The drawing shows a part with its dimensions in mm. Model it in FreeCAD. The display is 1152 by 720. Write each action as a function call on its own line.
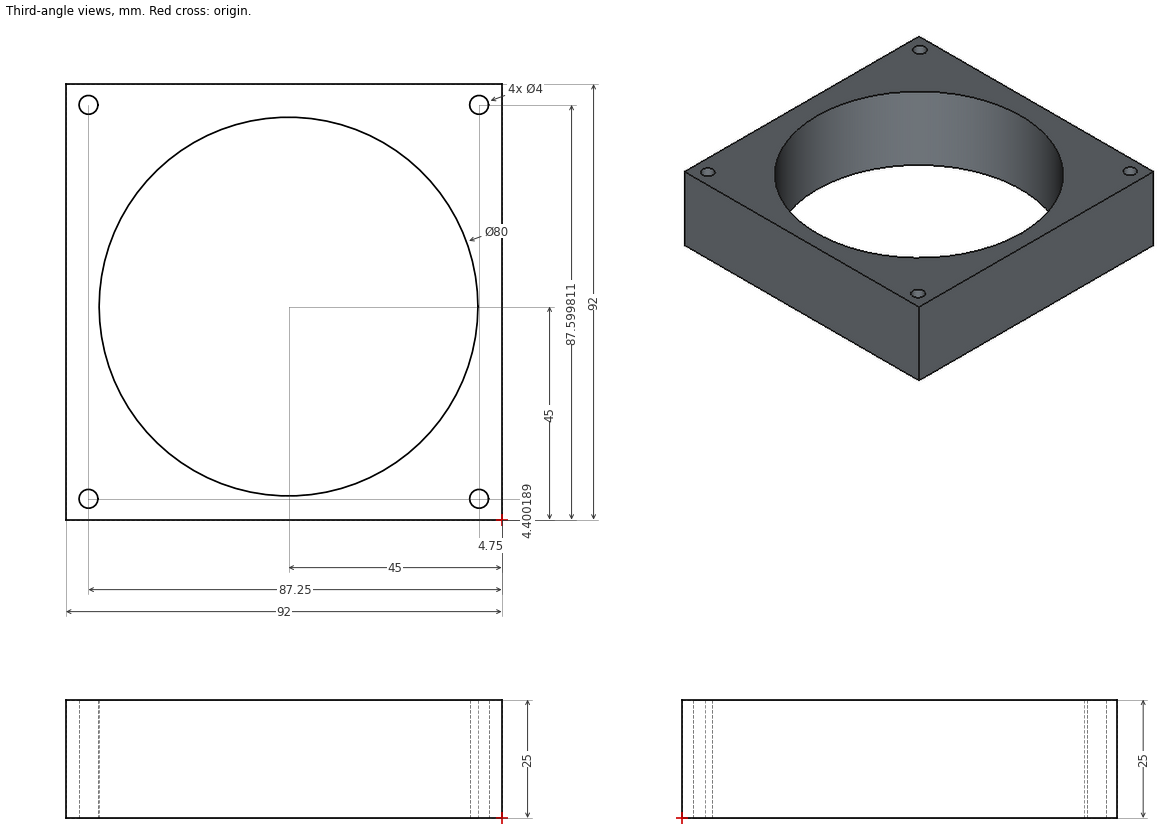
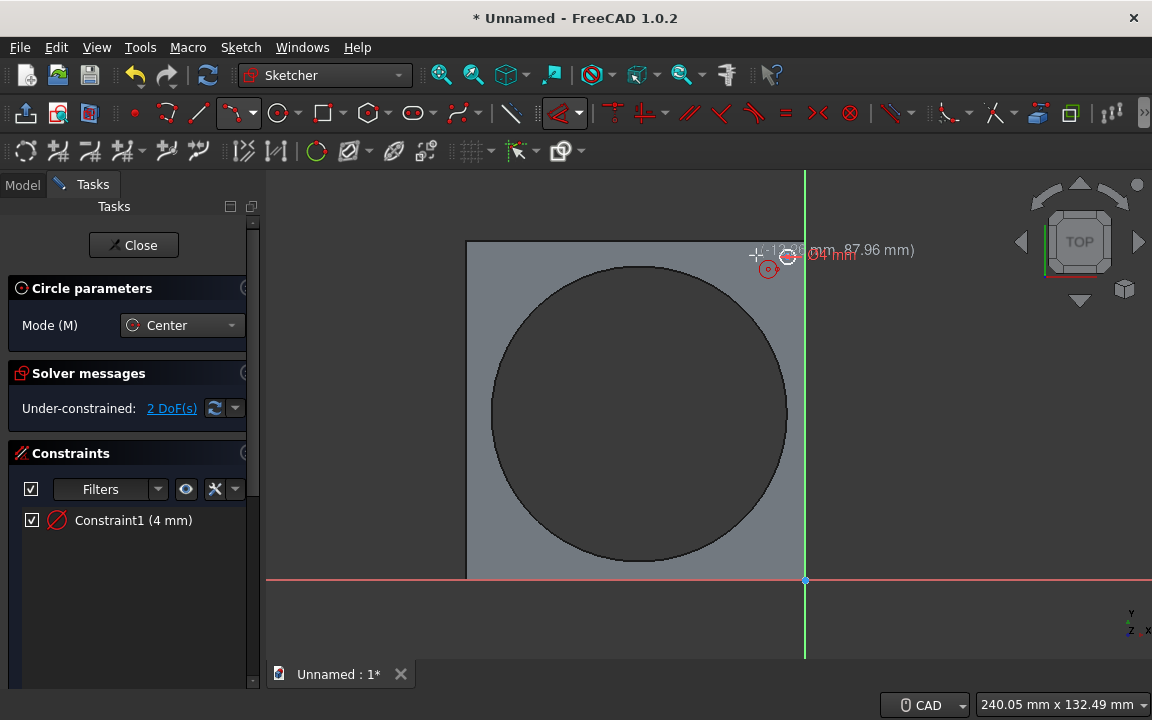
scroll(483, 257, up, 6)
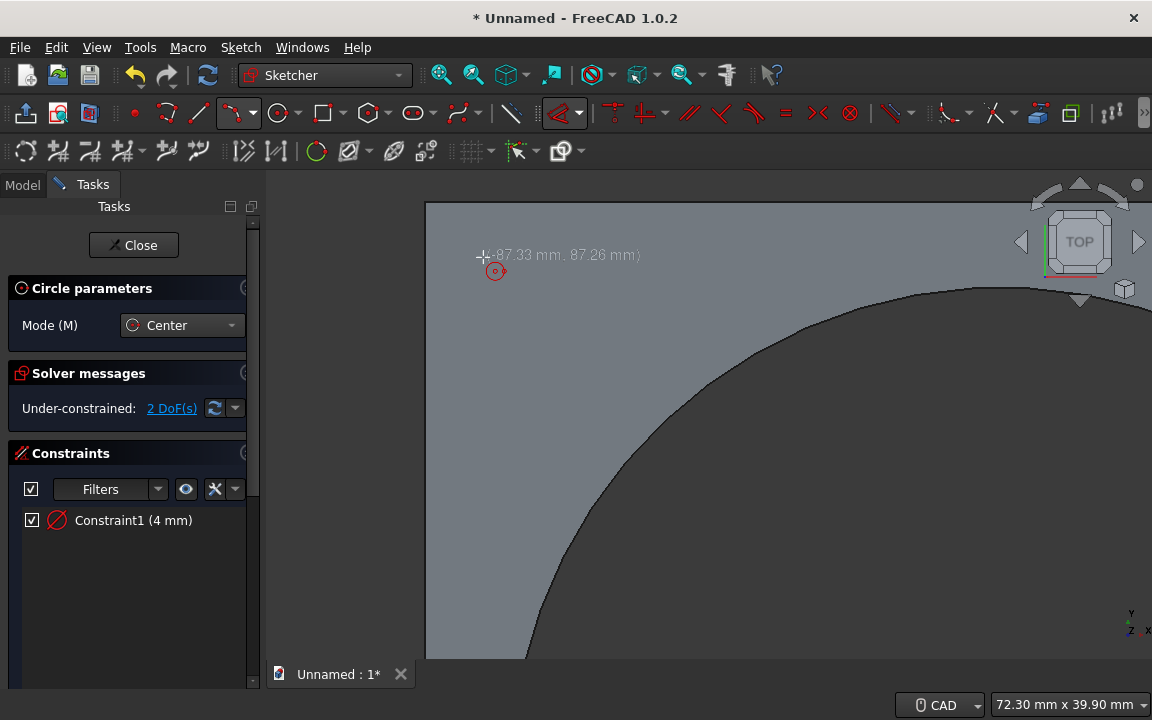
click(483, 256)
move(501, 238)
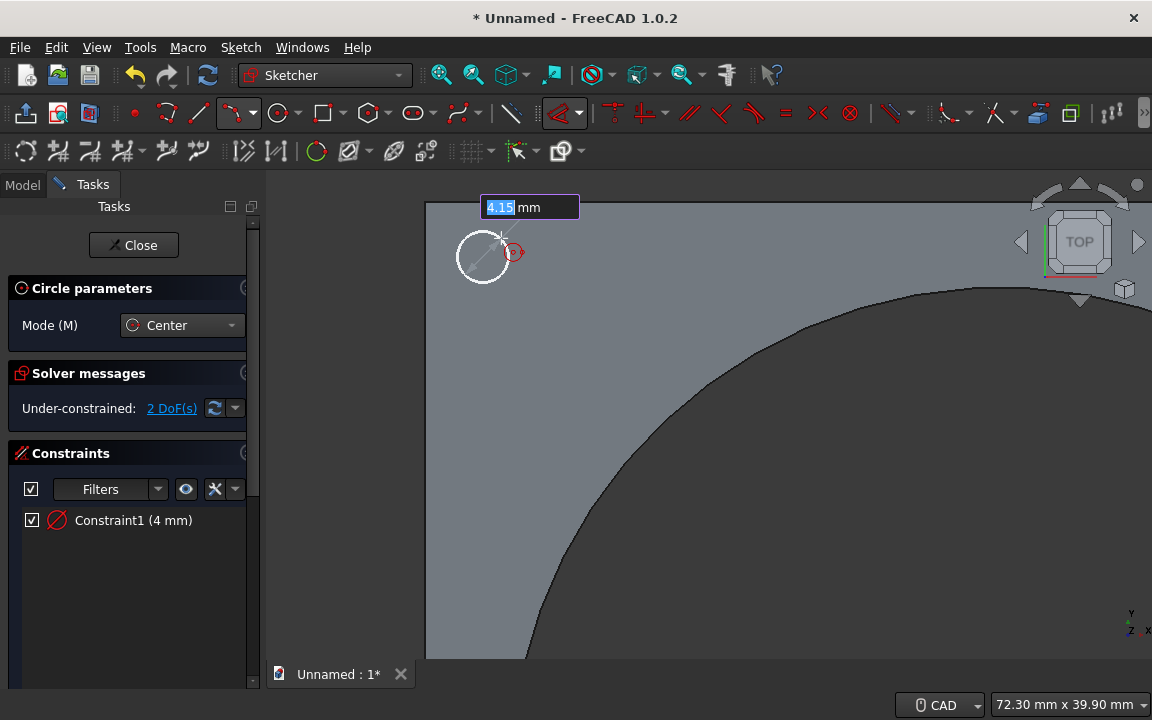
text(4)
key(Return)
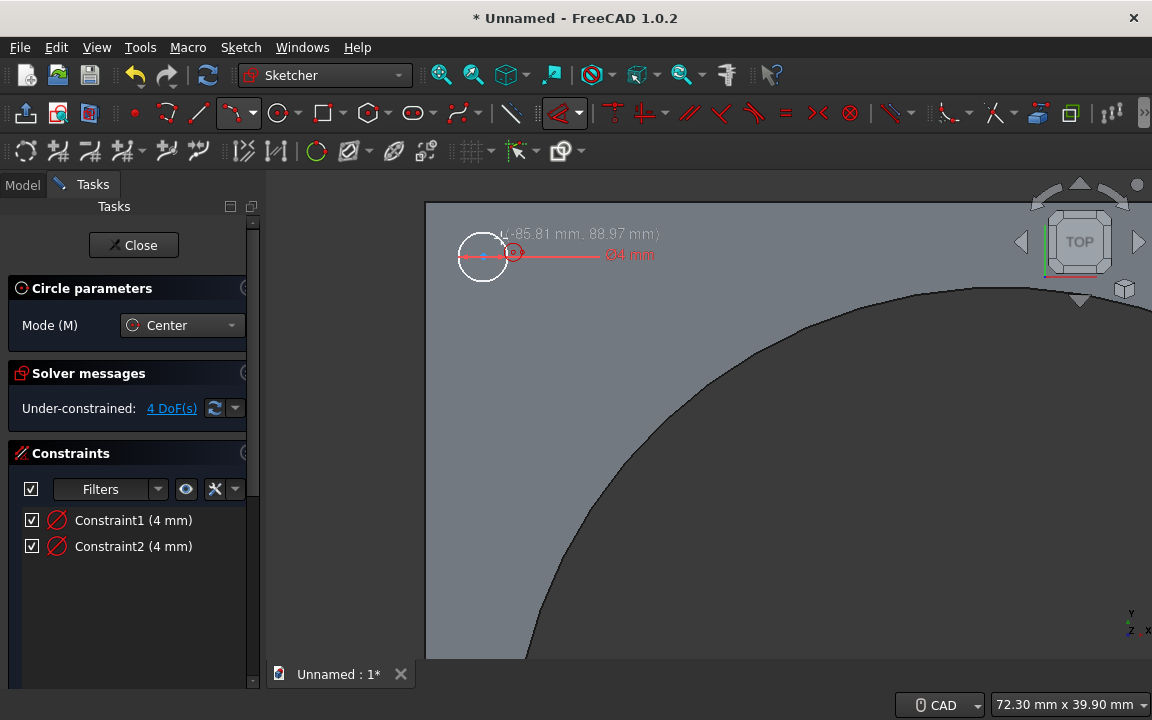
scroll(483, 257, down, 6)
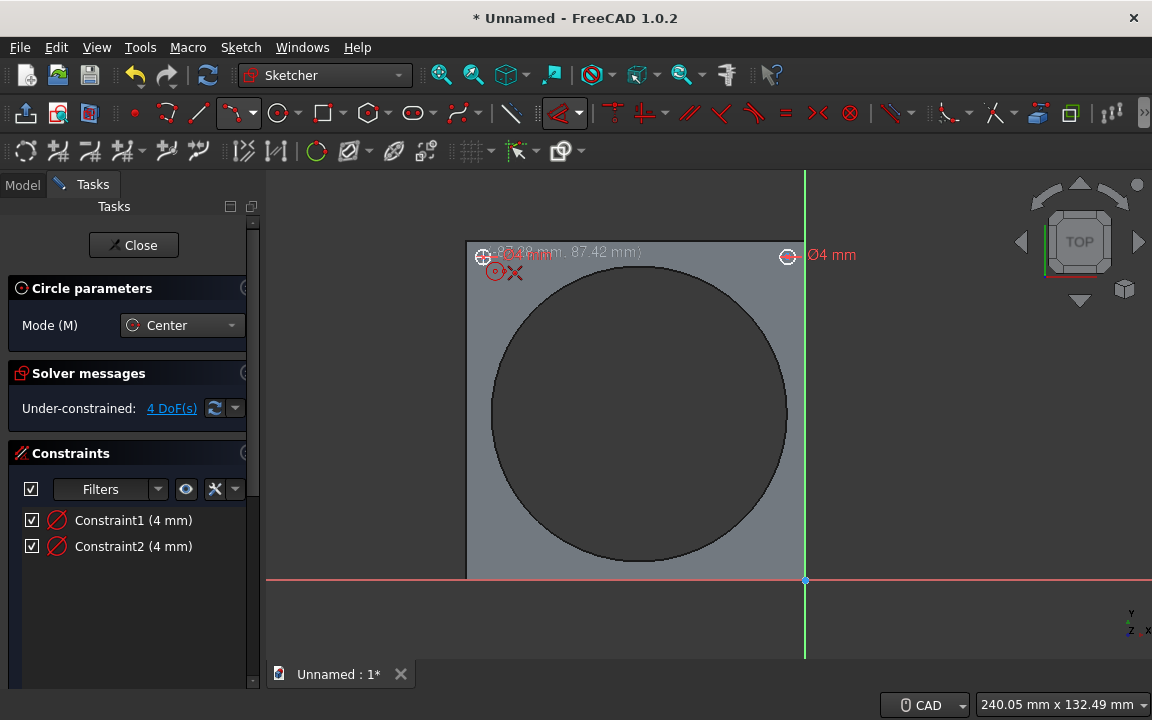
scroll(483, 564, up, 6)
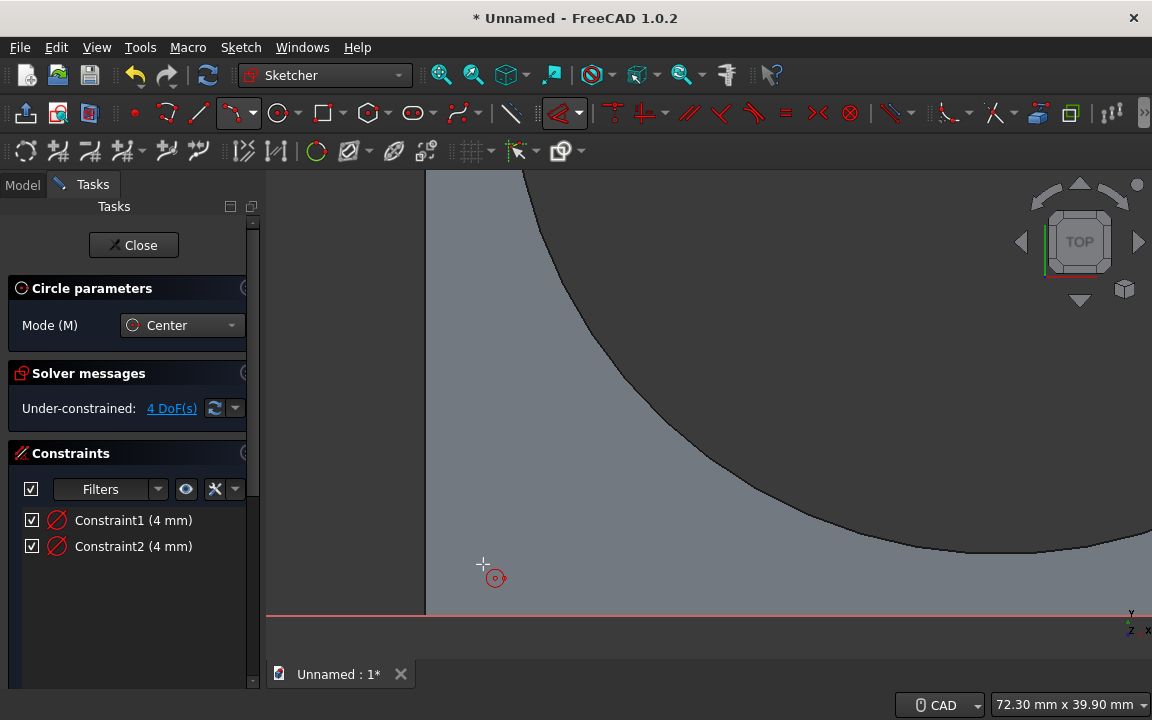
click(483, 562)
move(501, 544)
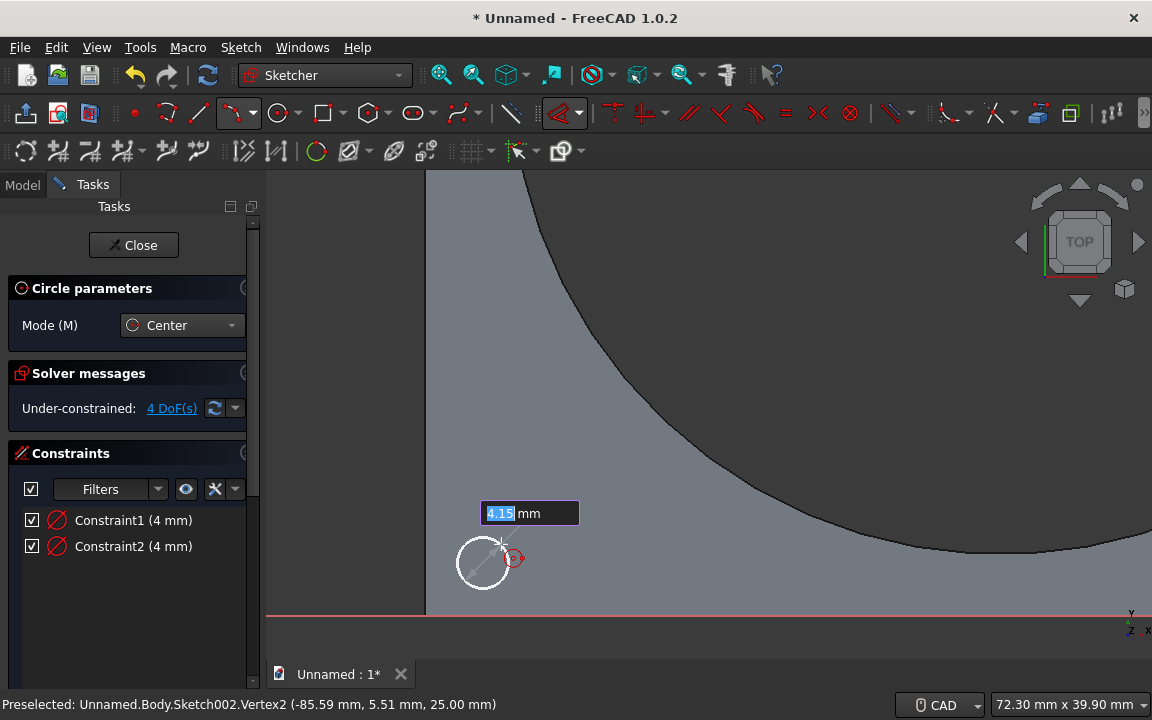
text(4)
key(Return)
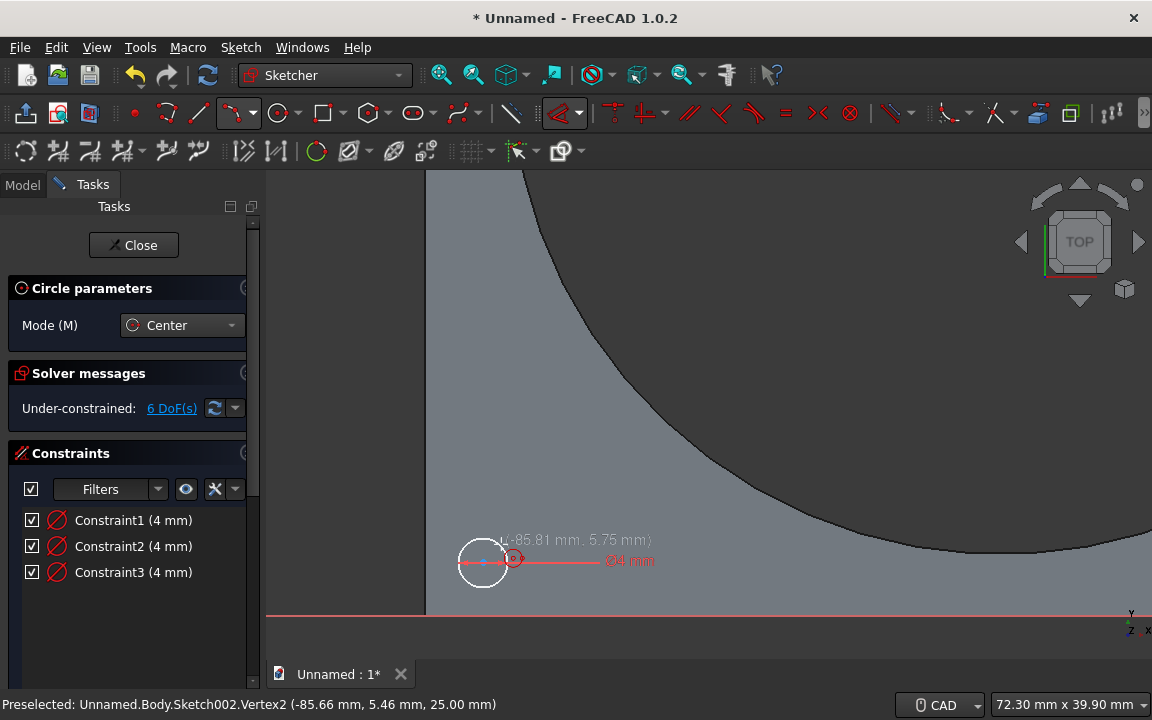
scroll(483, 564, down, 6)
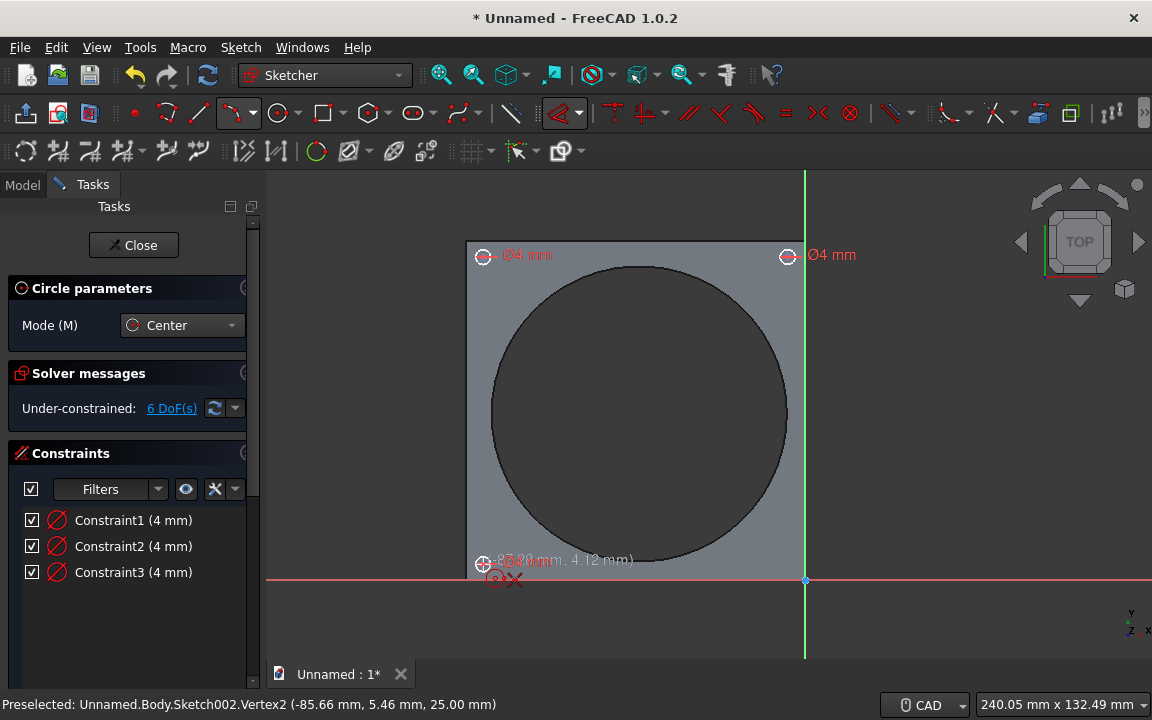
scroll(788, 564, up, 6)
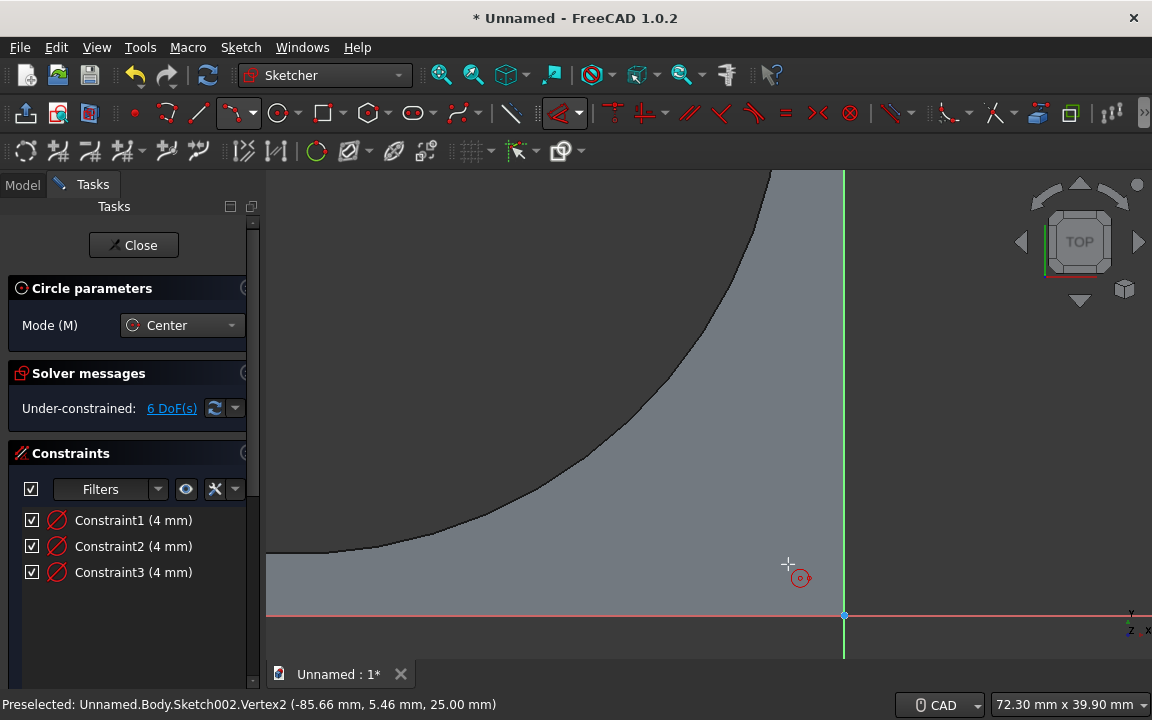
click(786, 562)
move(803, 544)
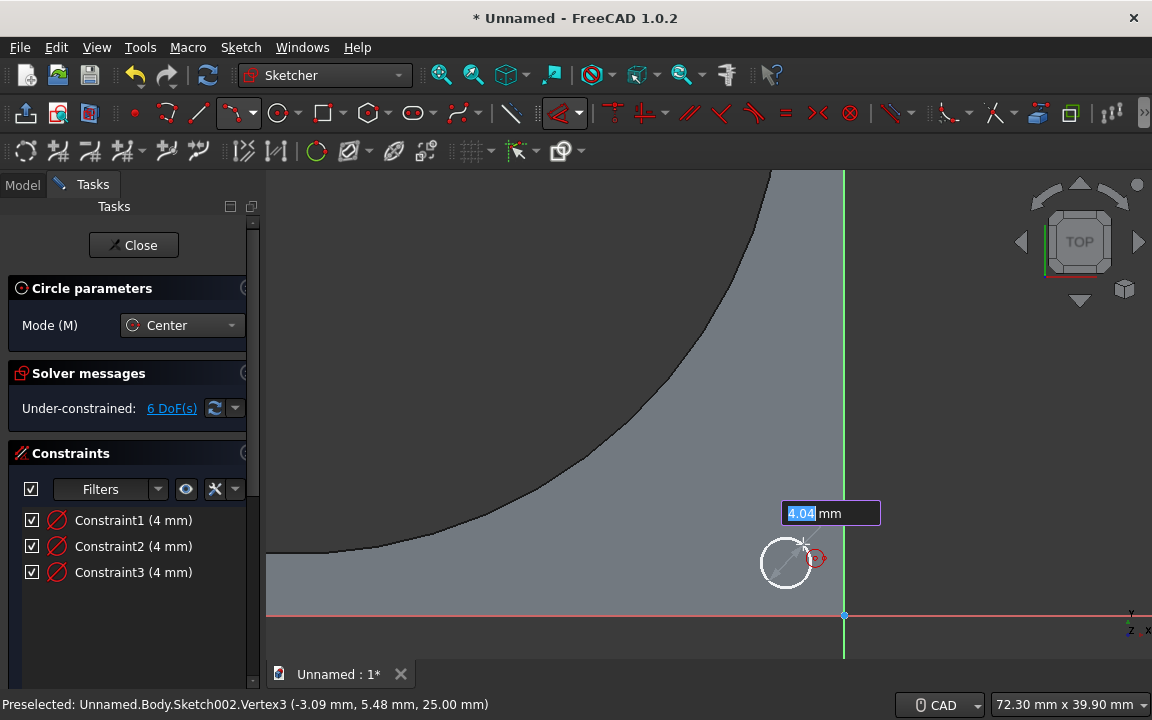
text(4)
key(Return)
key(Escape)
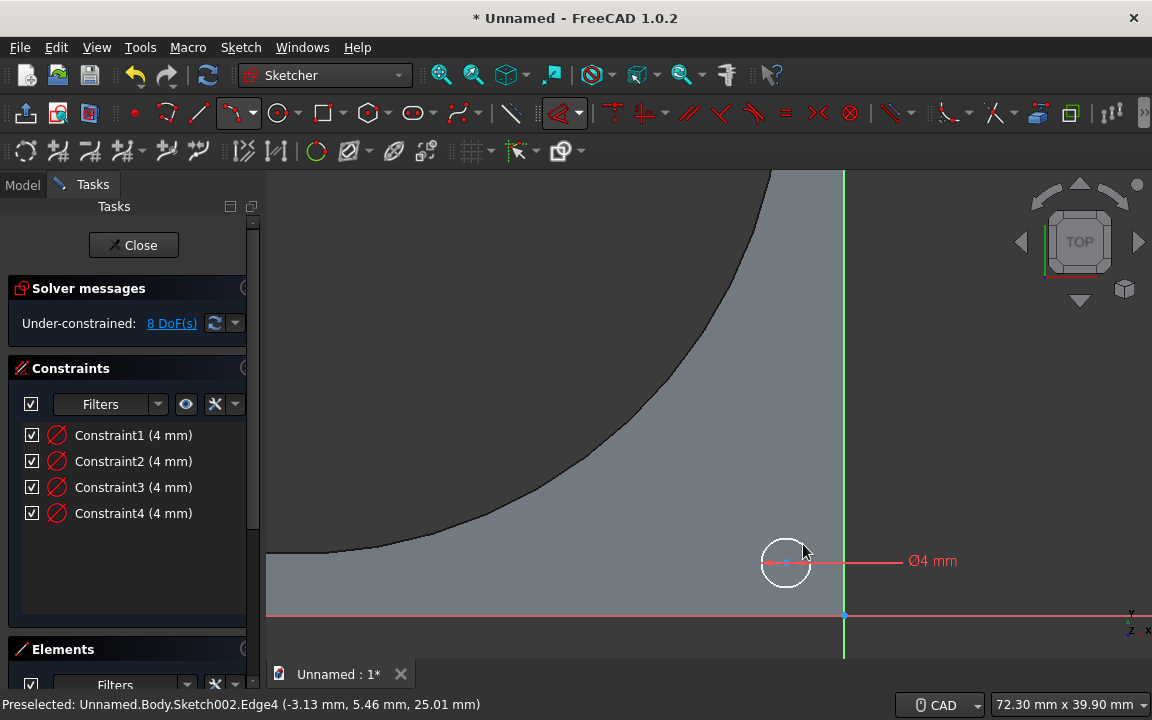
scroll(788, 564, down, 6)